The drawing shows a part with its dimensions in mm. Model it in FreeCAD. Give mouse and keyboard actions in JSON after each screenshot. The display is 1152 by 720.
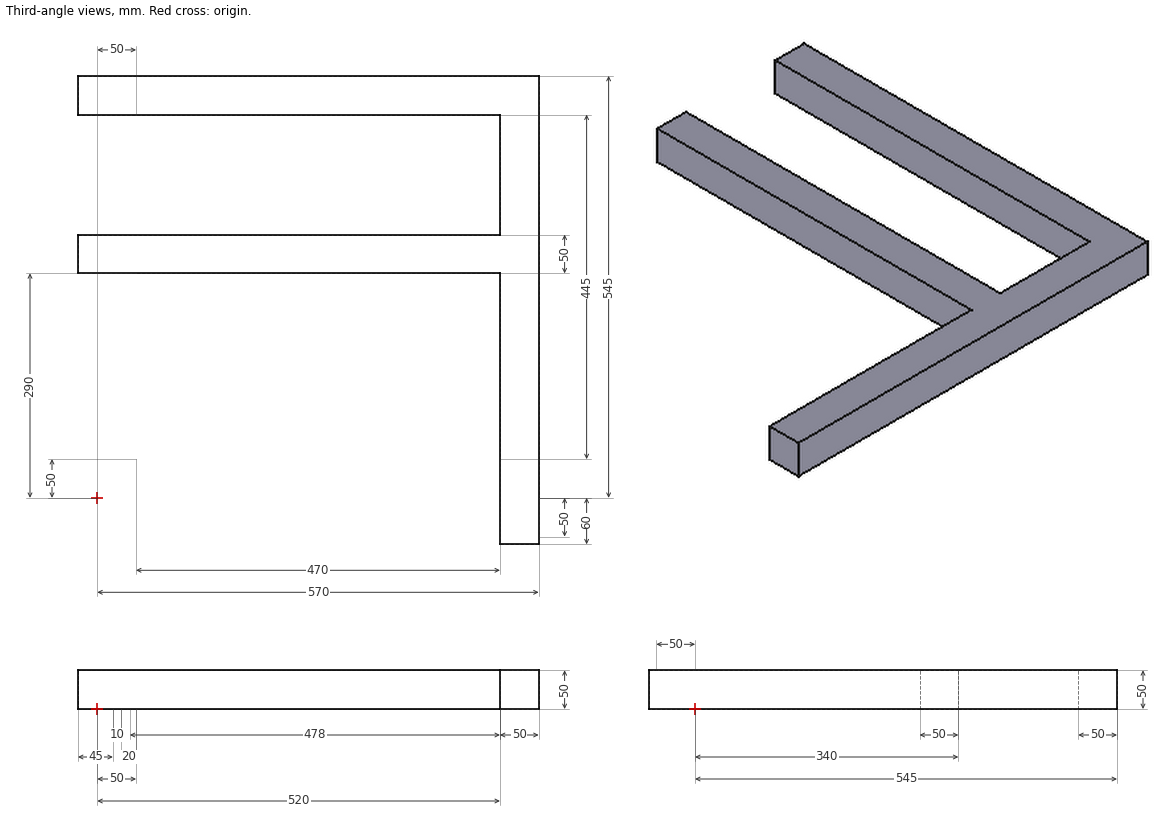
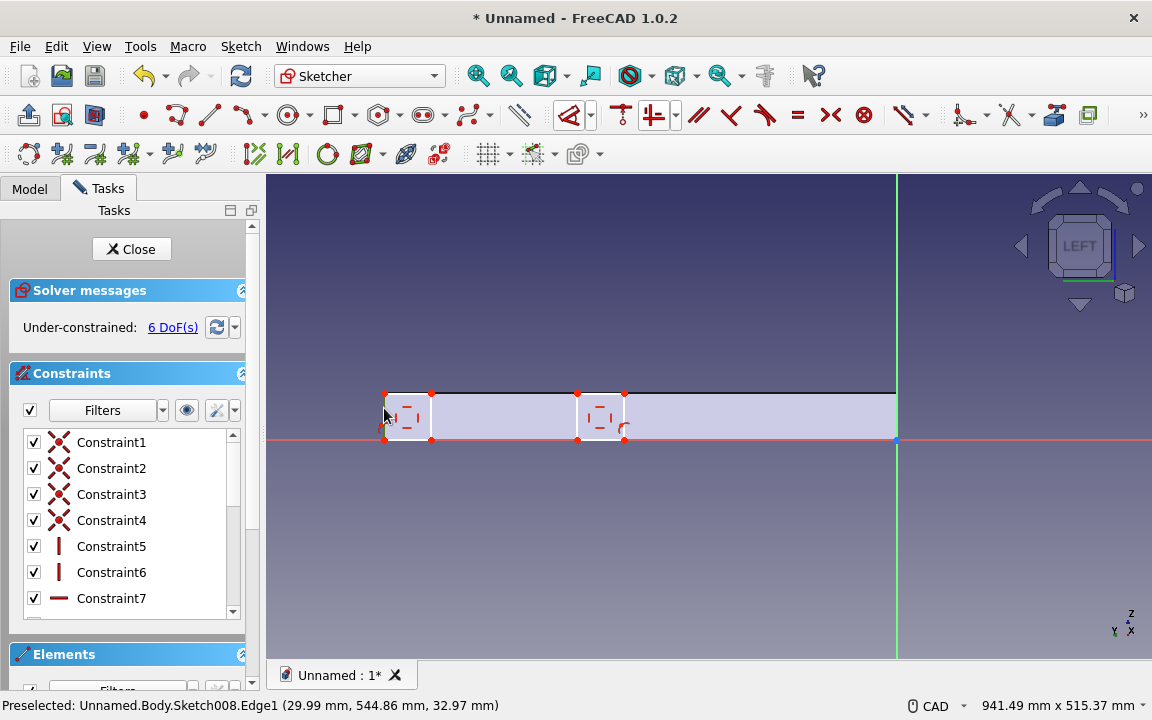
{"action": "key", "text": "i"}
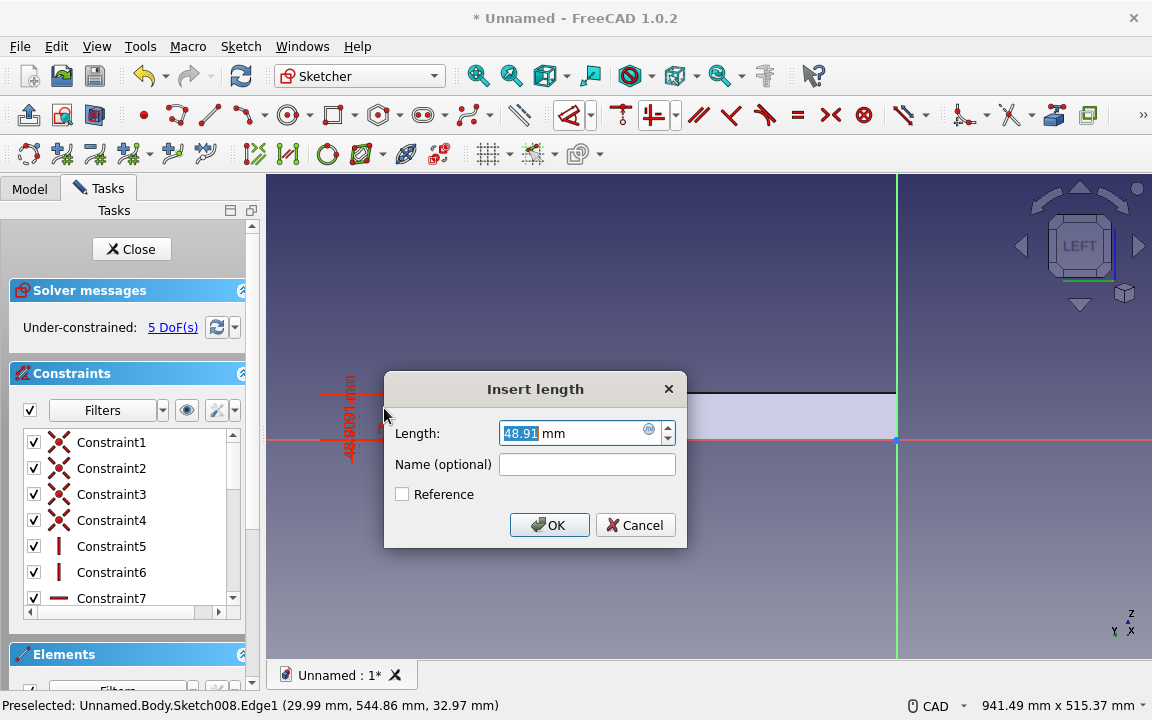
{"action": "type", "text": "50"}
{"action": "key", "text": "Return"}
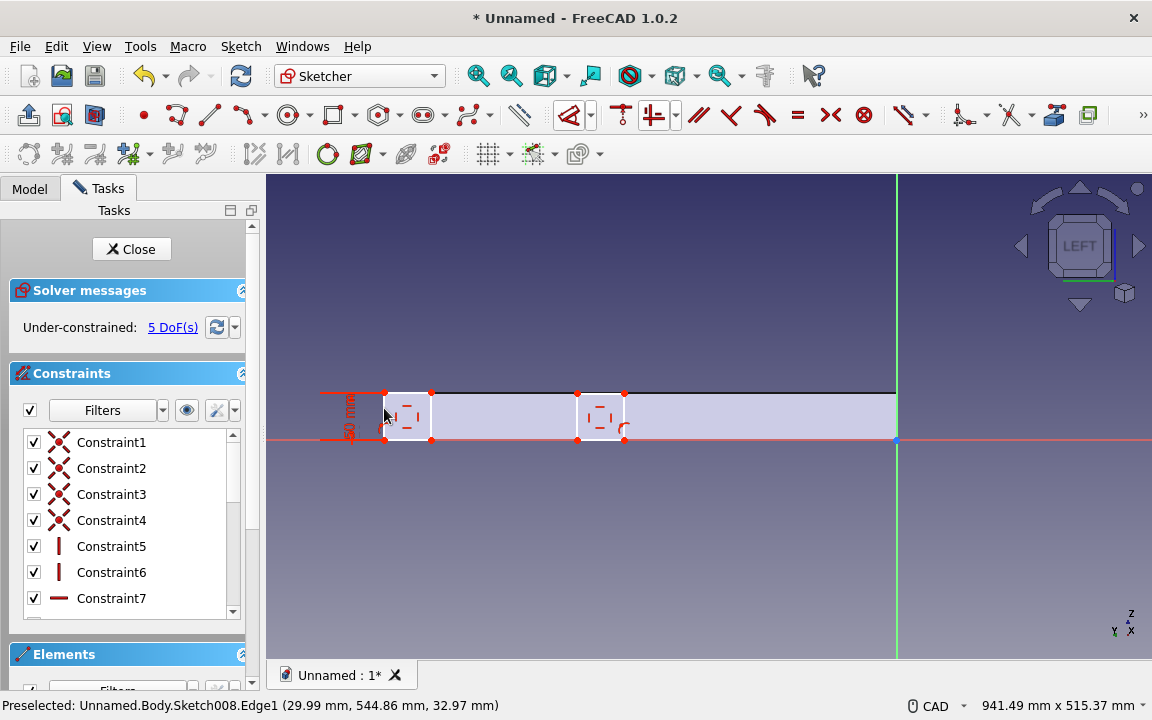
{"action": "left_click", "coordinate": [398, 440]}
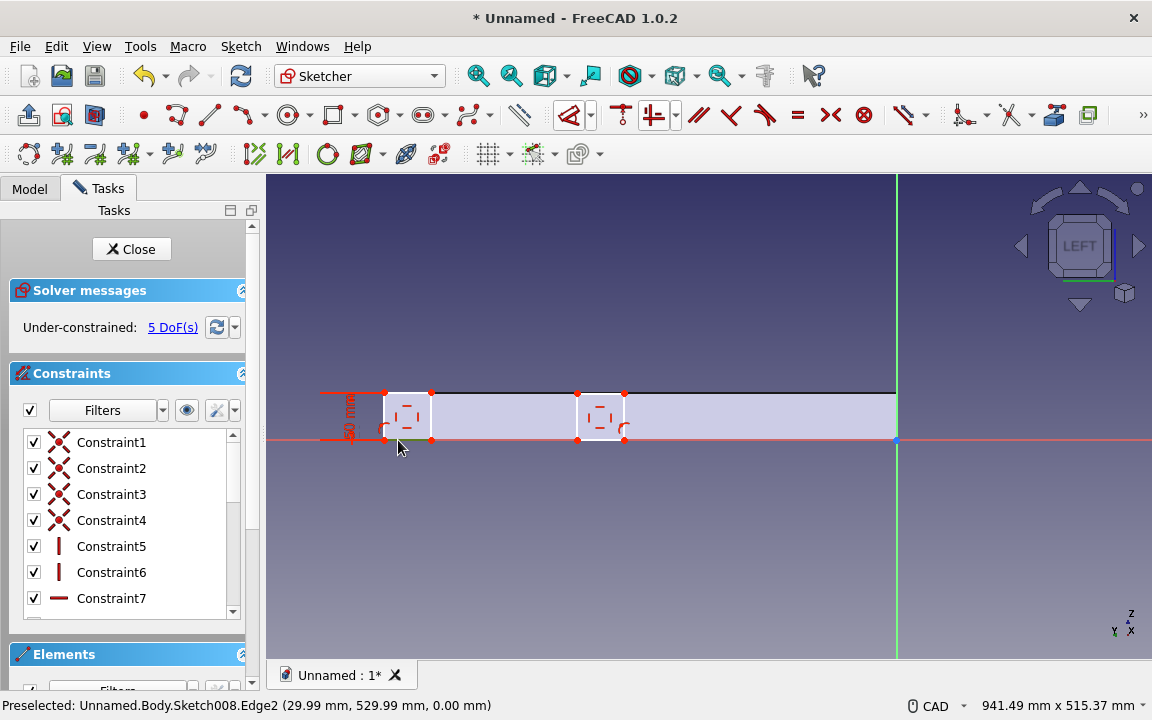
{"action": "key", "text": "l"}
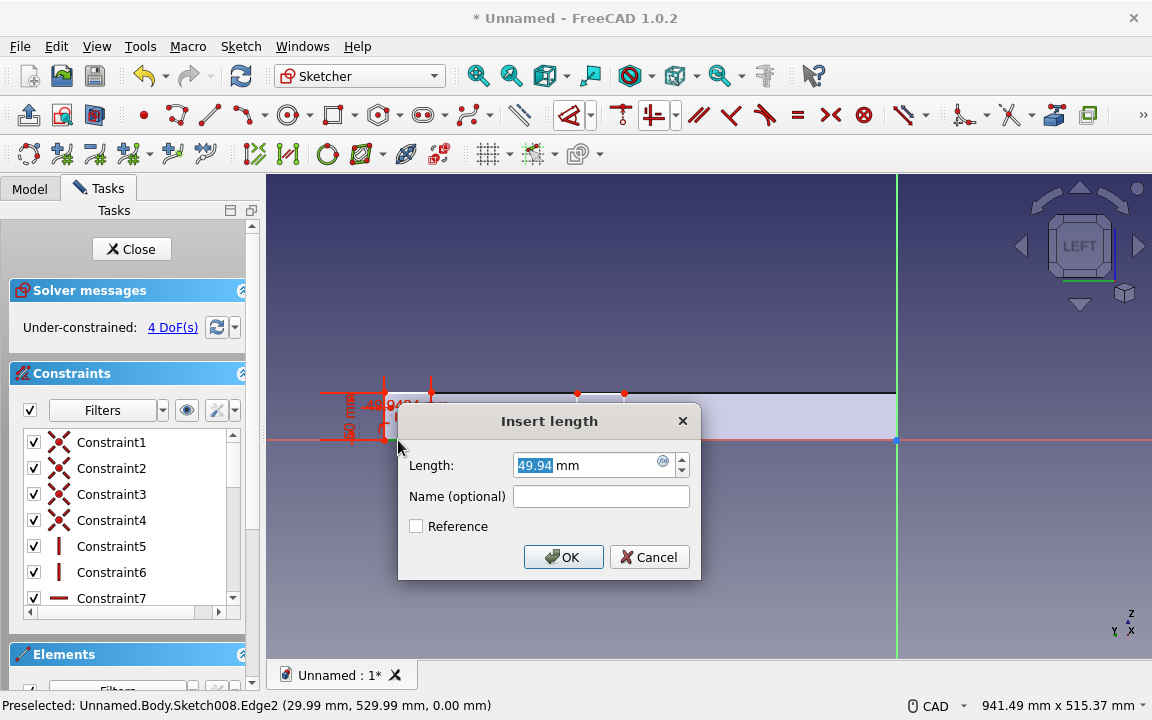
{"action": "type", "text": "50"}
{"action": "key", "text": "Return"}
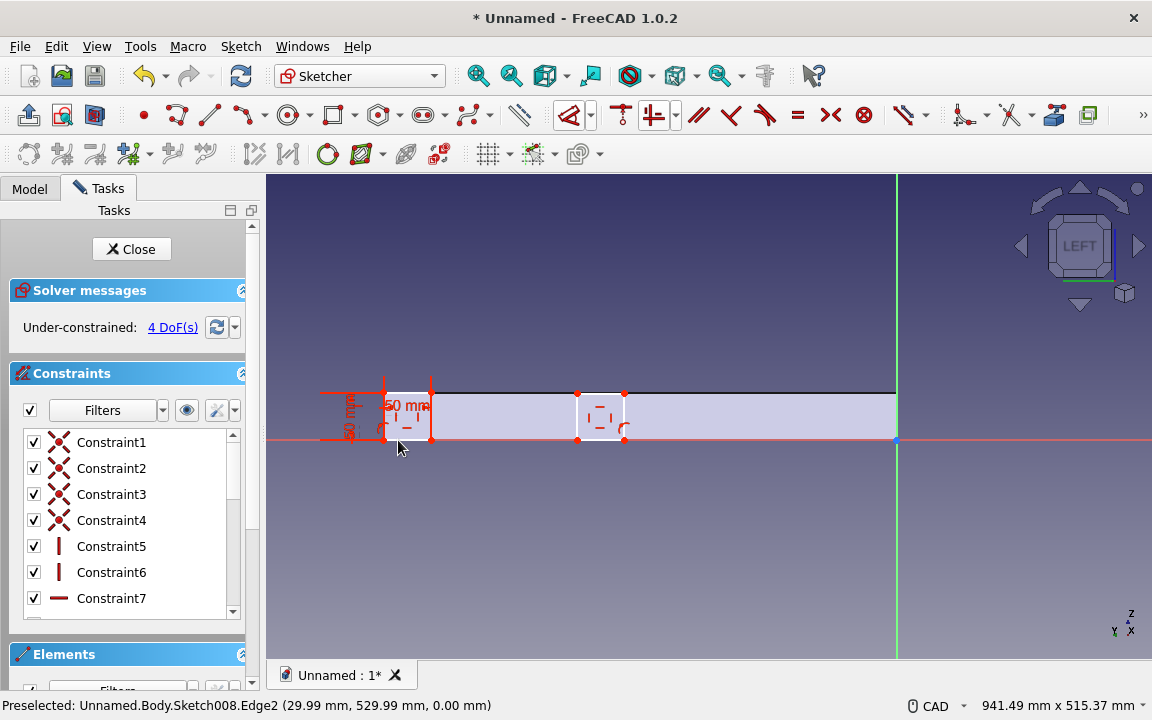
{"action": "left_click", "coordinate": [577, 408]}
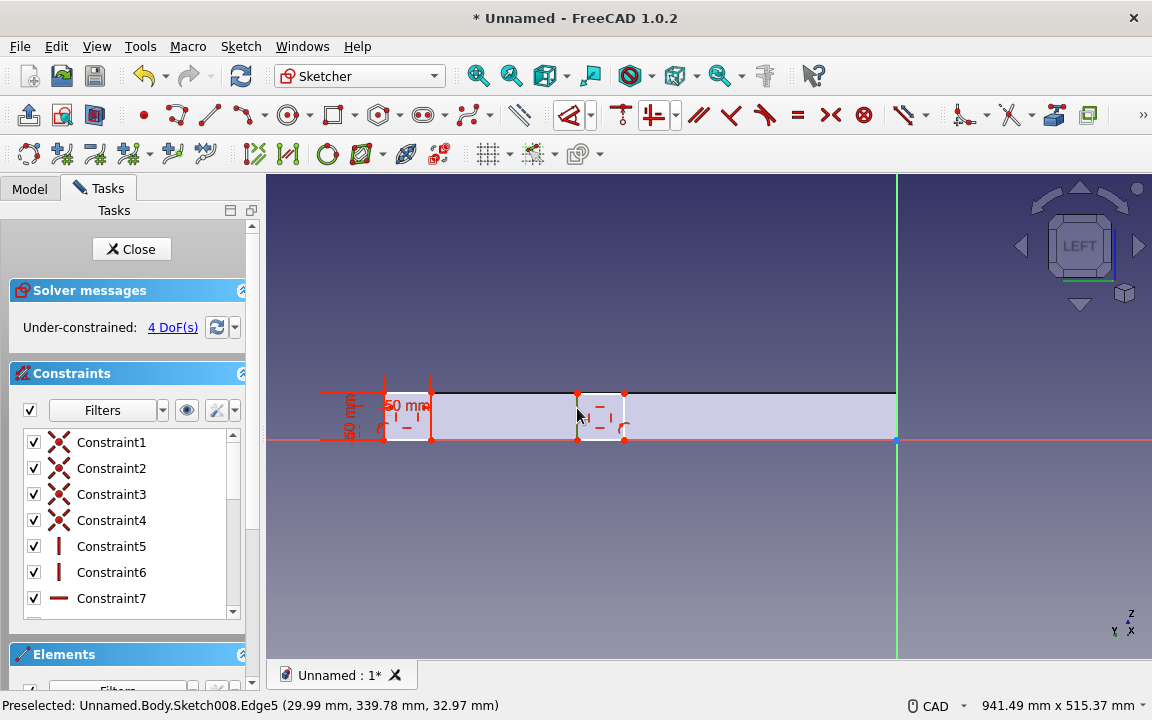
{"action": "key", "text": "i"}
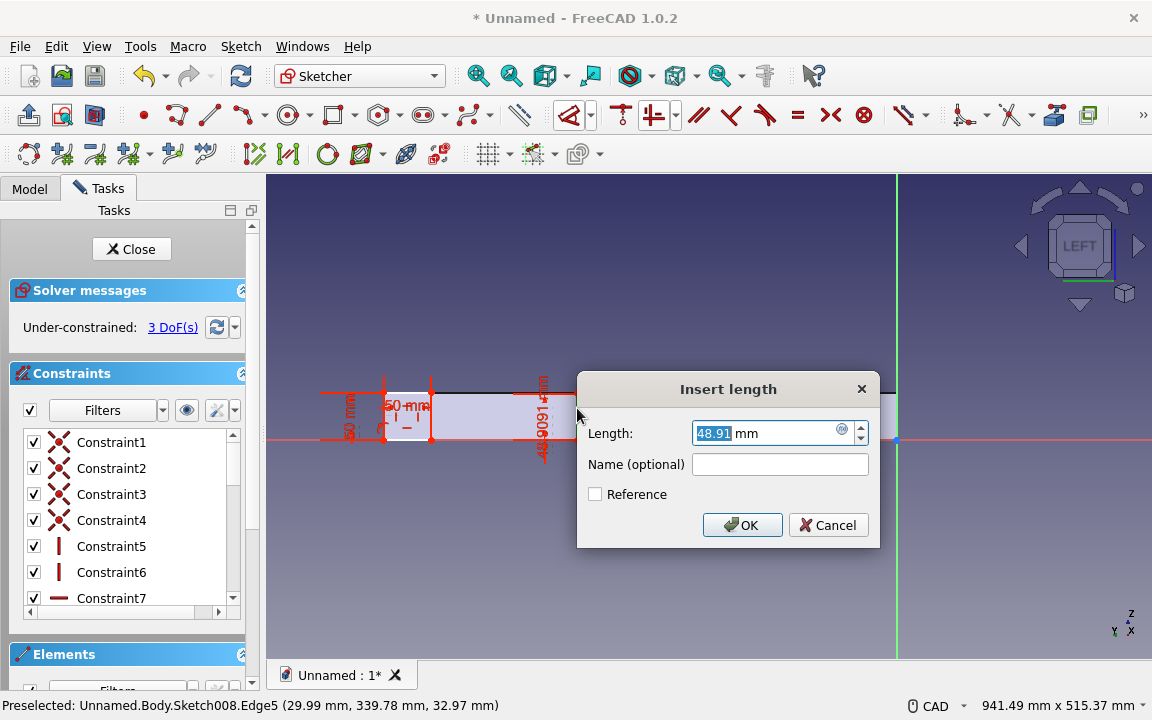
{"action": "type", "text": "50"}
{"action": "key", "text": "Return"}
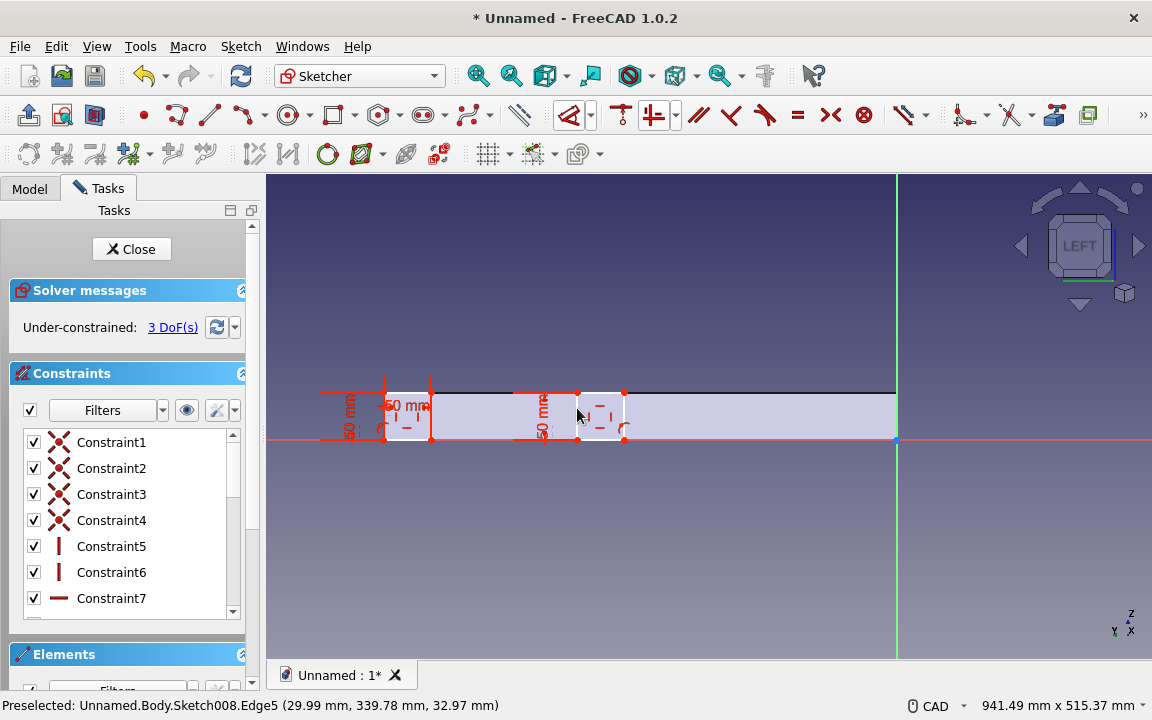
{"action": "left_click", "coordinate": [591, 440]}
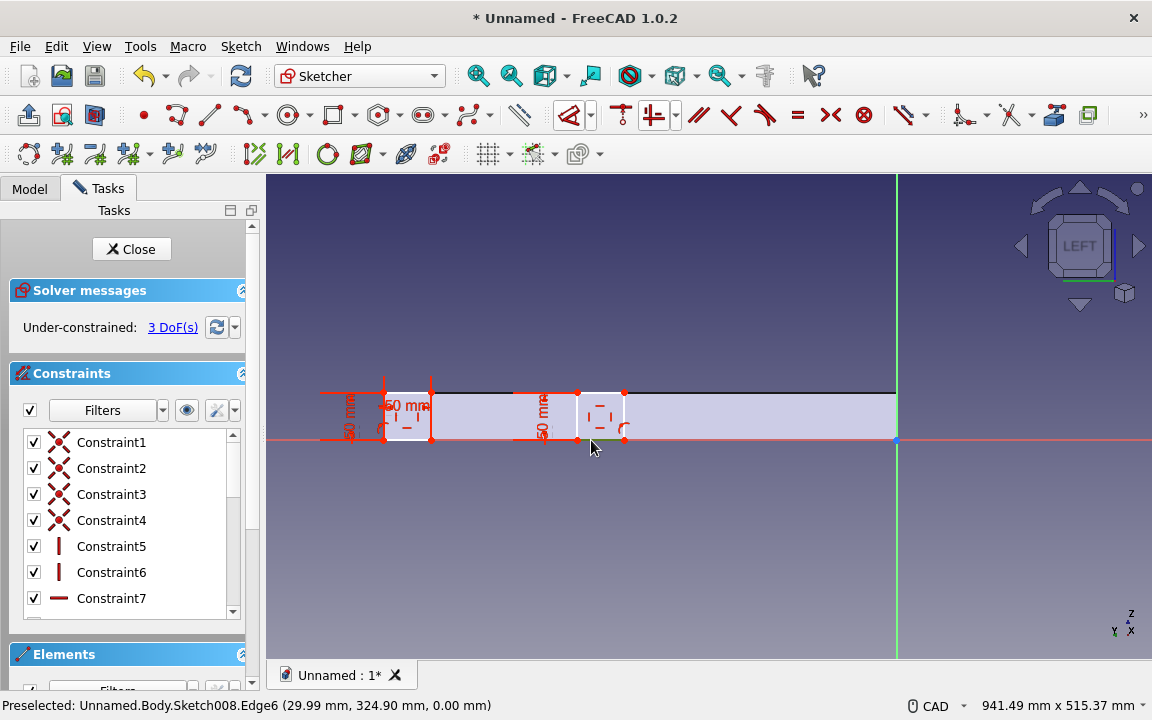
{"action": "key", "text": "l"}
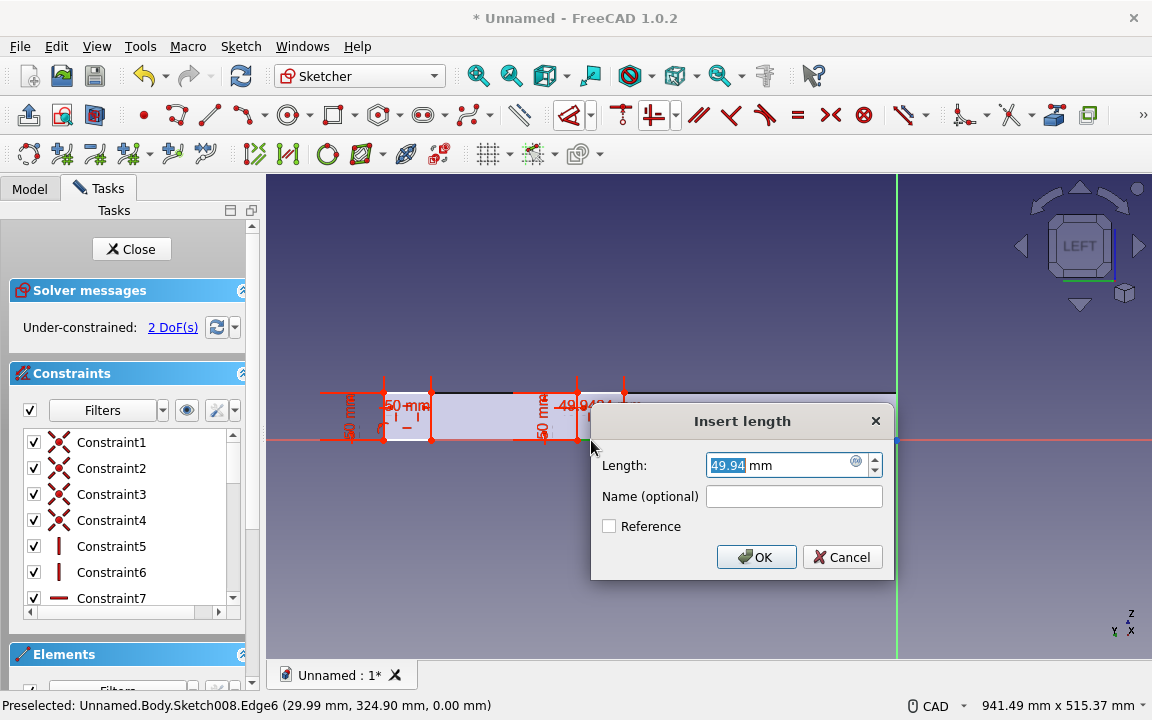
{"action": "type", "text": "50"}
{"action": "key", "text": "Return"}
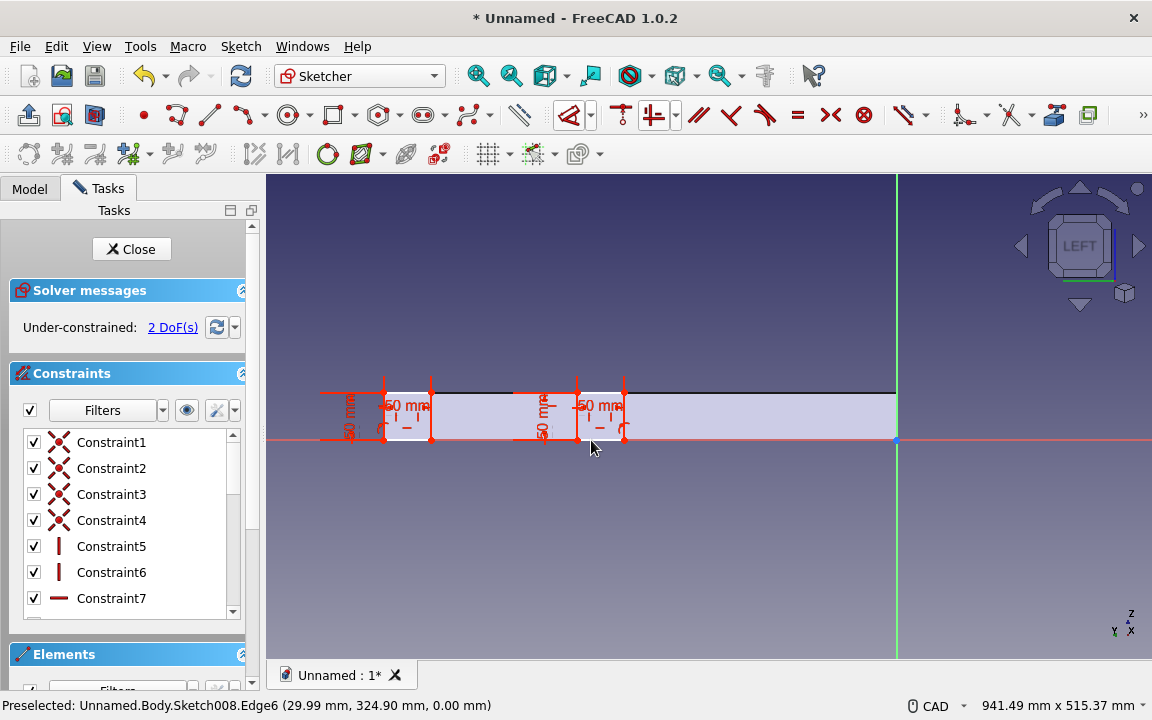
{"action": "left_click", "coordinate": [384, 393]}